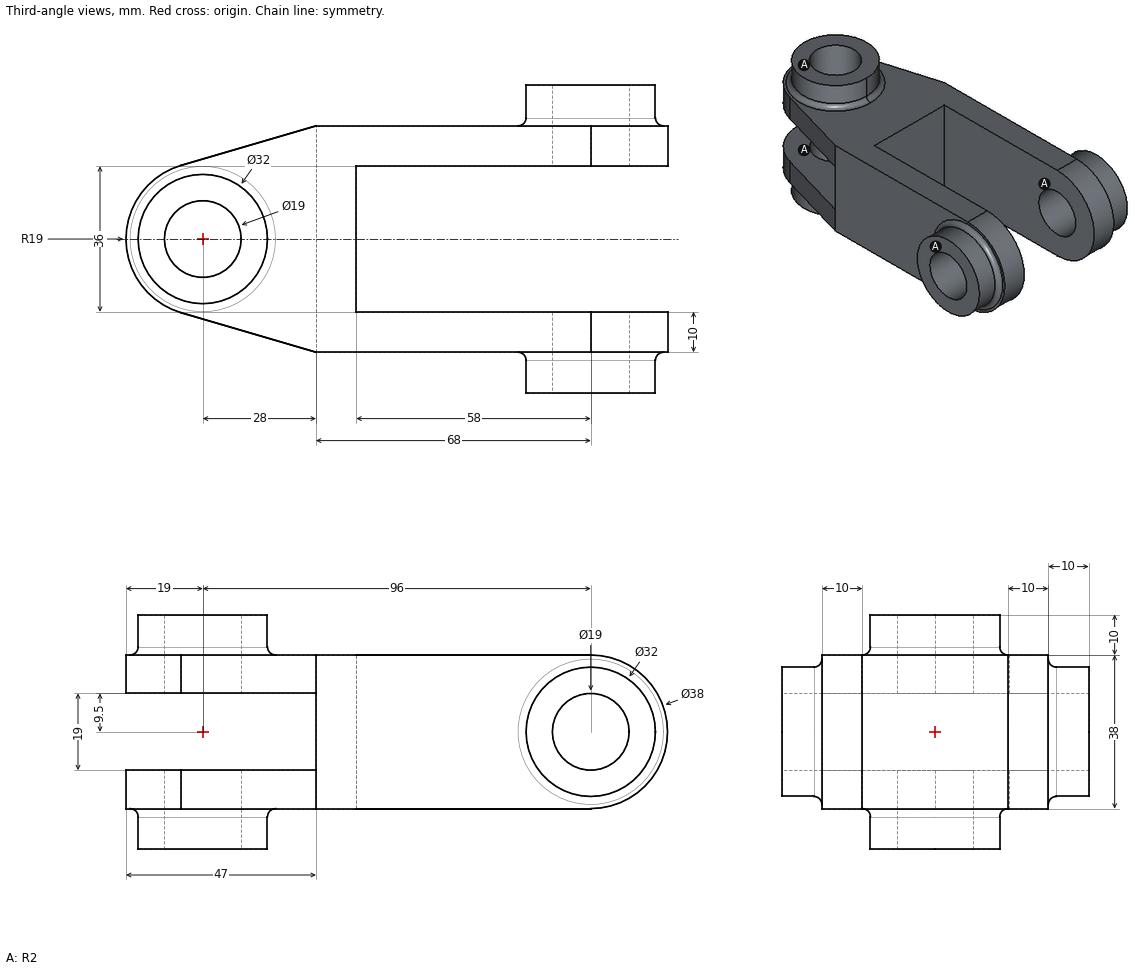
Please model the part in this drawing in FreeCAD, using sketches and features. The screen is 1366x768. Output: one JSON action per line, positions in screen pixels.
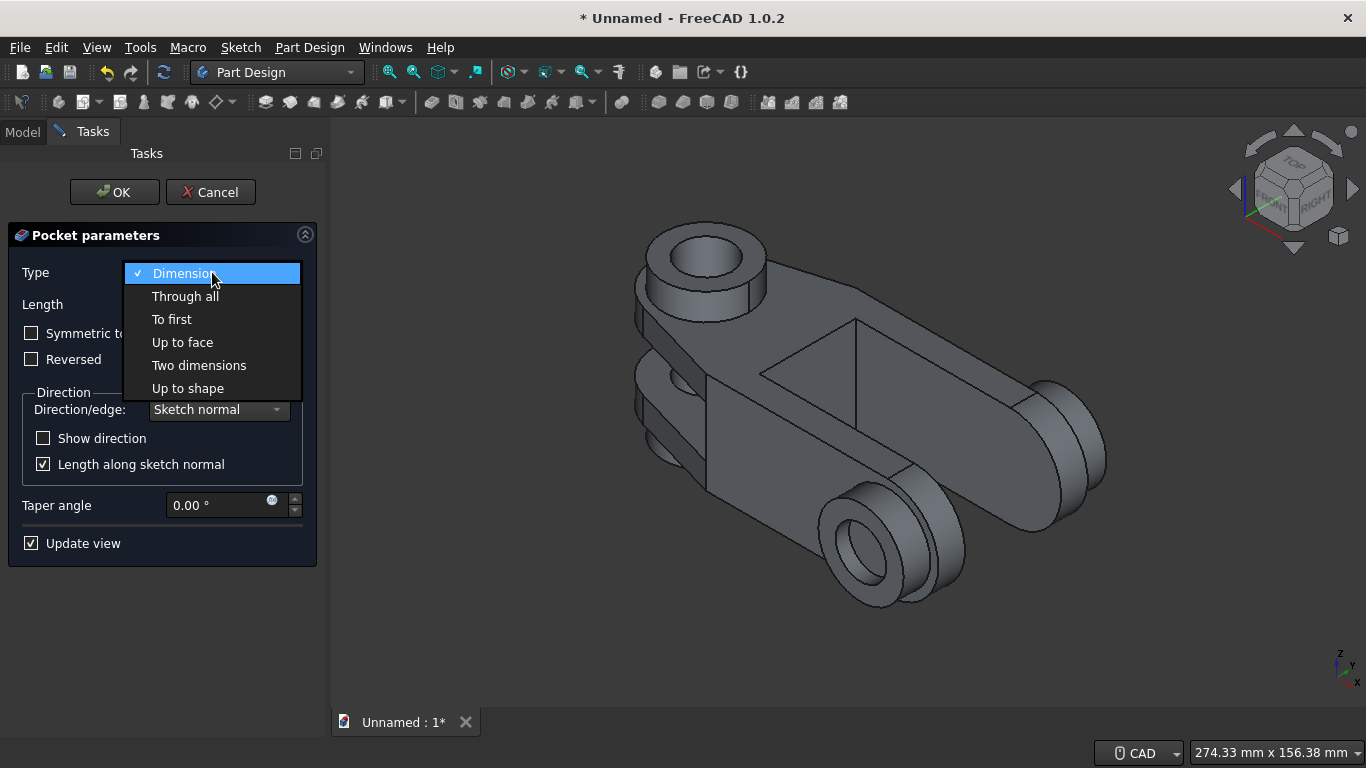
{"action": "left_click", "coordinate": [212, 296]}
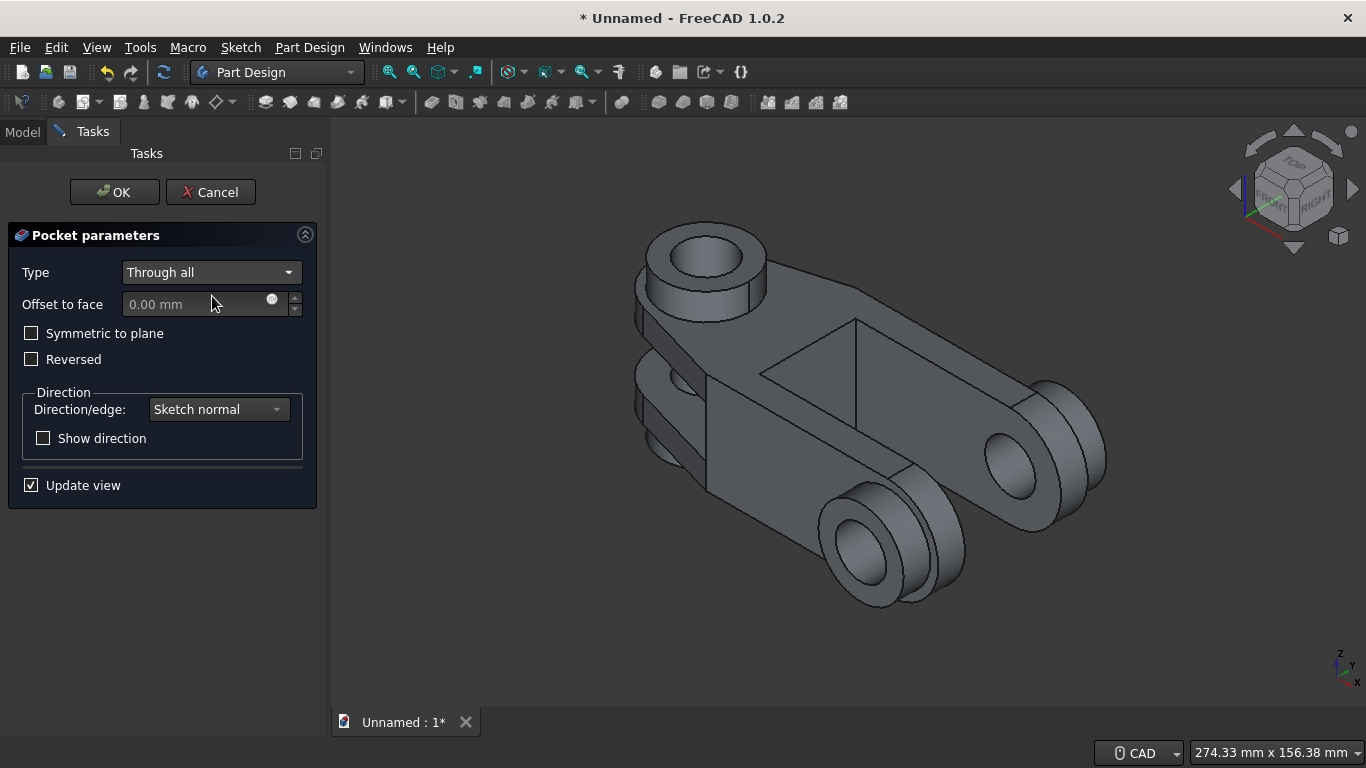
{"action": "left_click", "coordinate": [115, 192]}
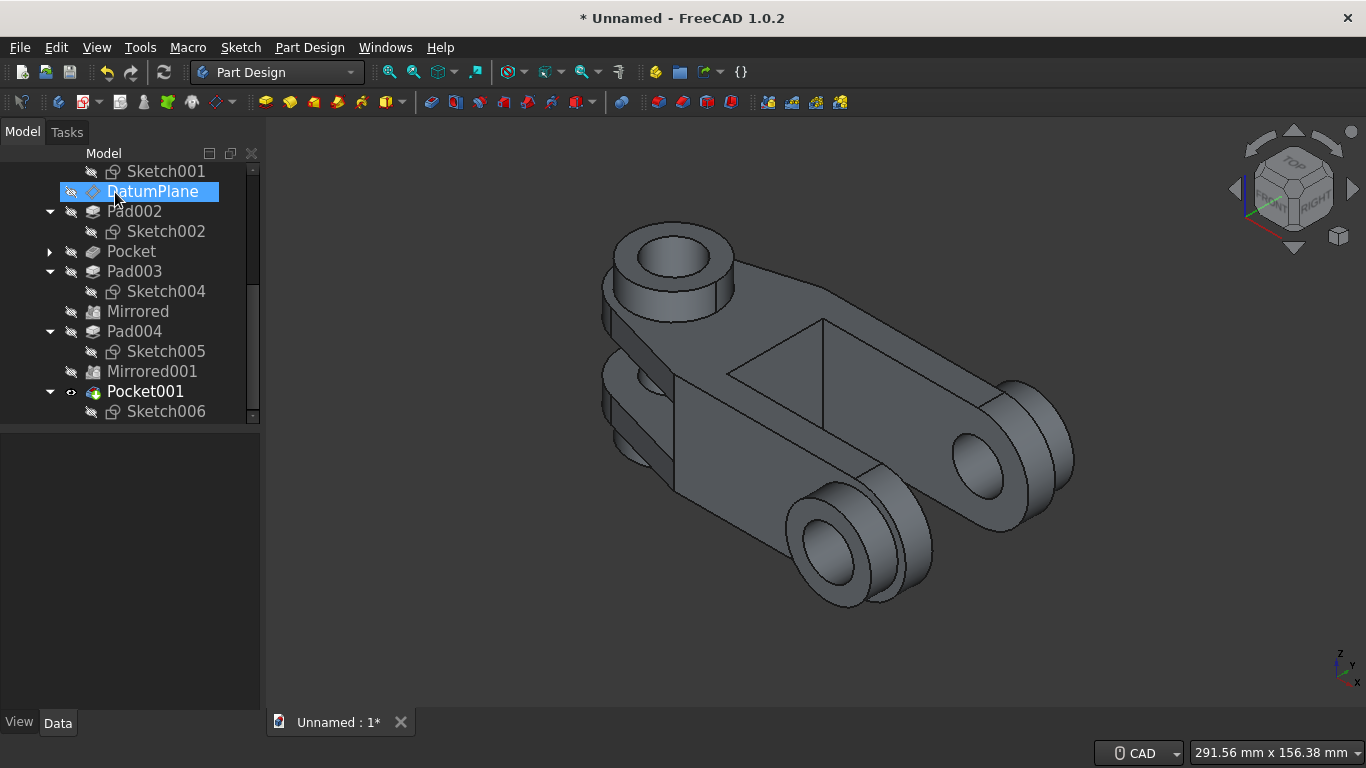
{"action": "key", "text": "2"}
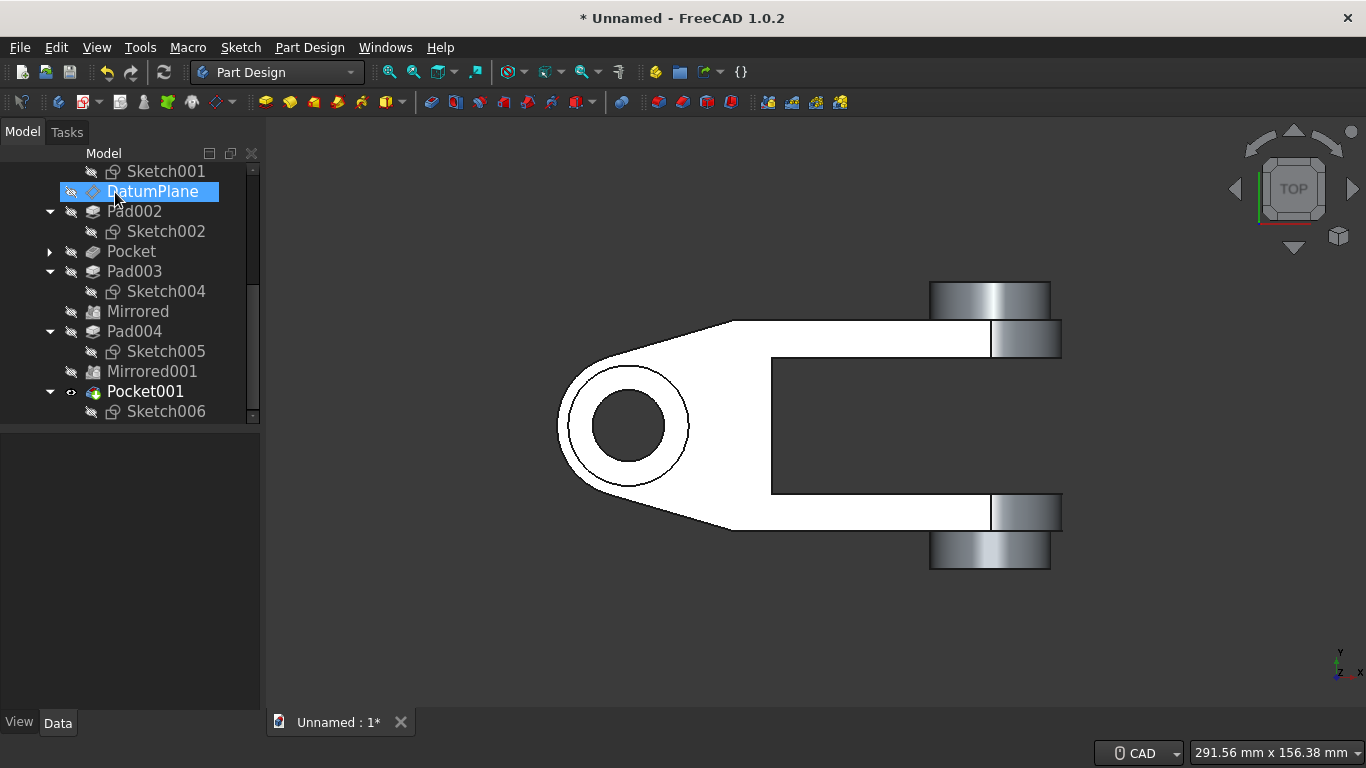
{"action": "key", "text": "0"}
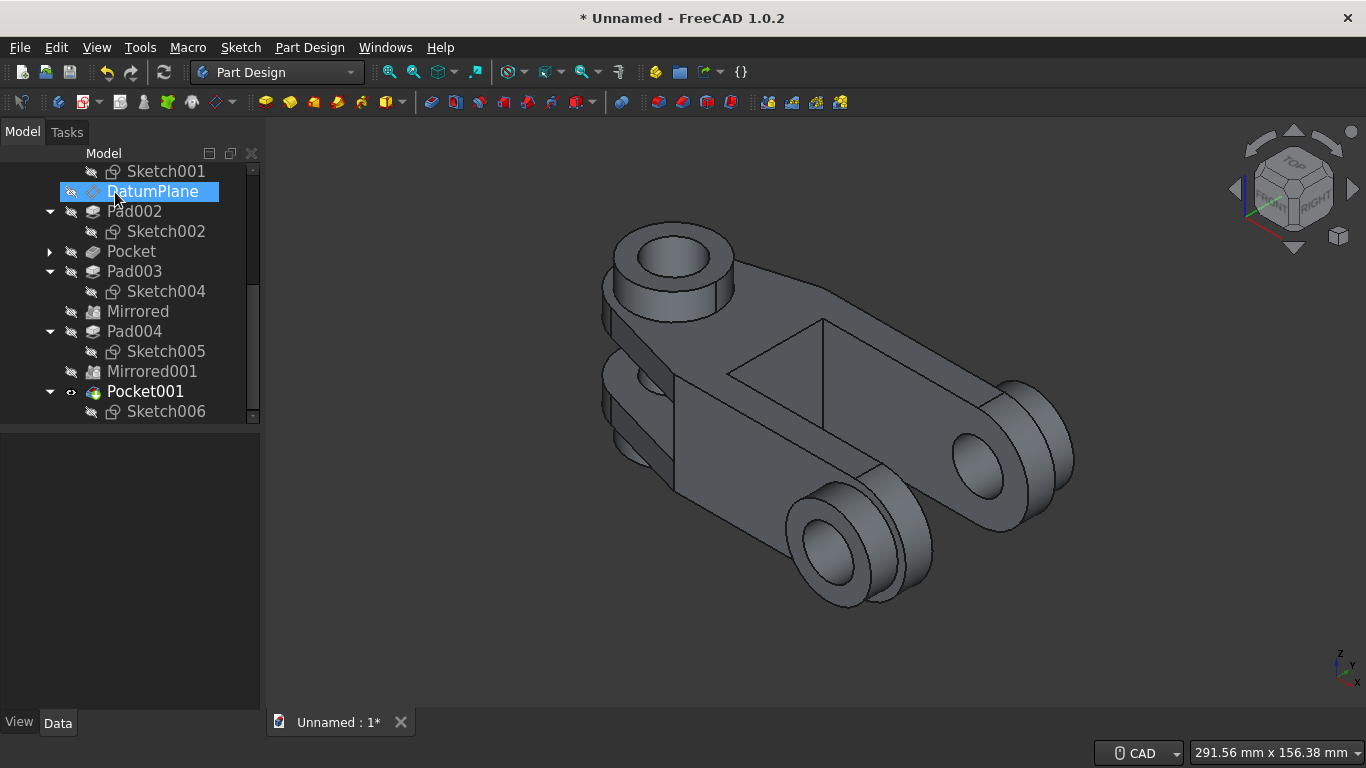
{"action": "key", "text": "1"}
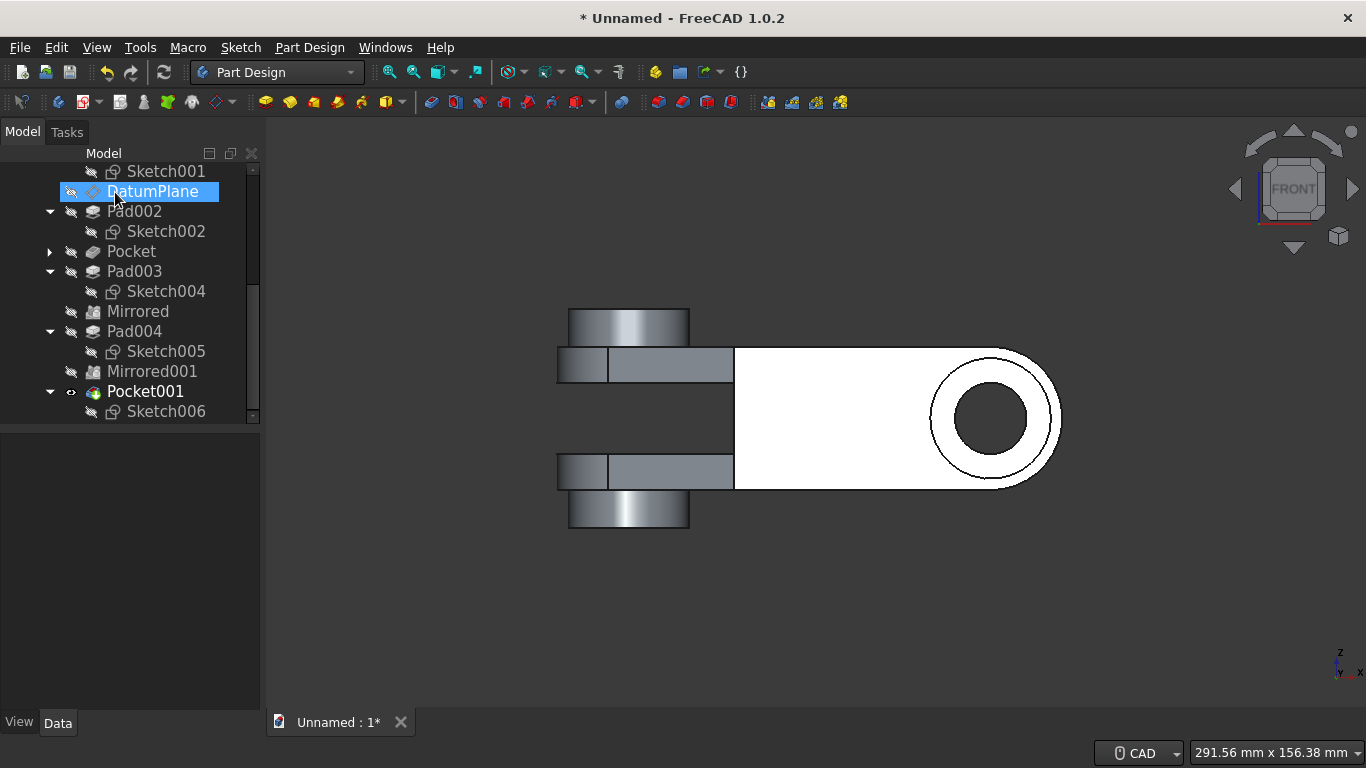
{"action": "key", "text": "3"}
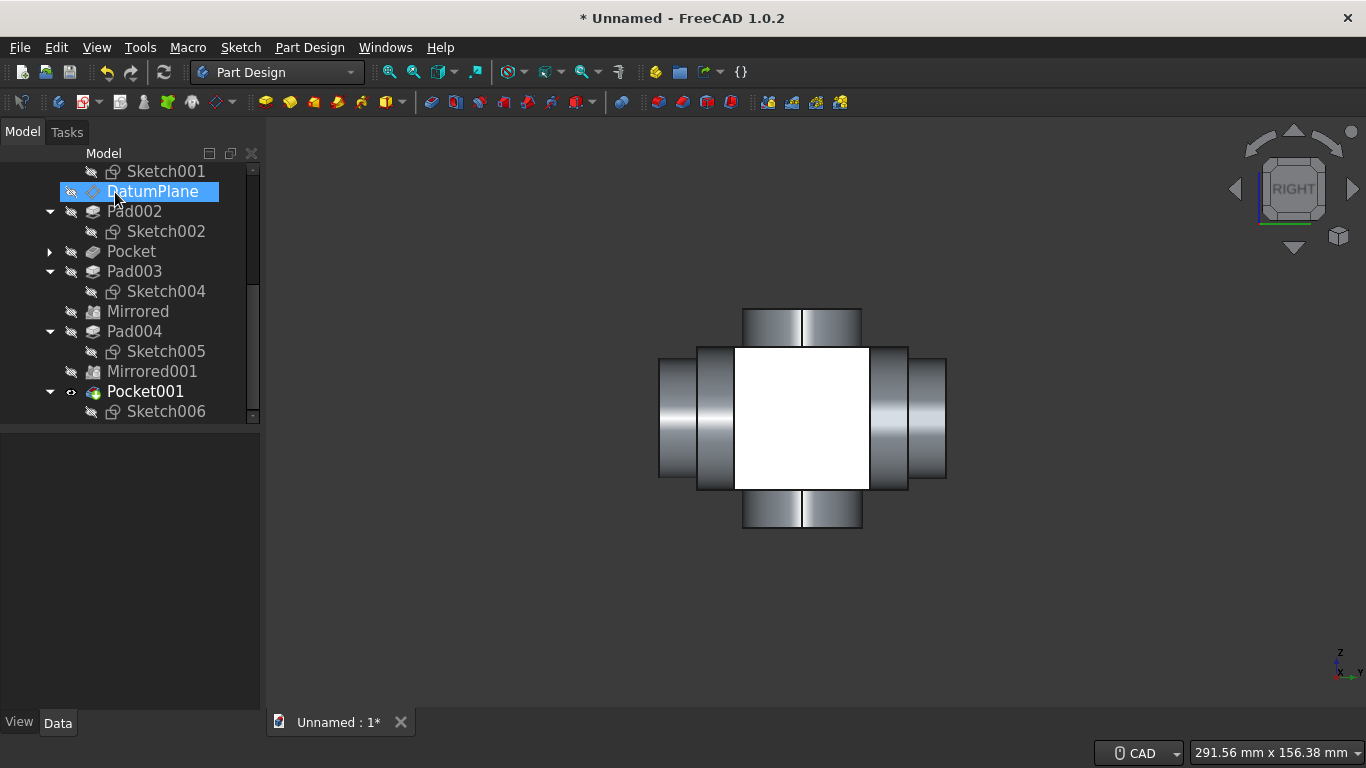
{"action": "left_click", "coordinate": [390, 72]}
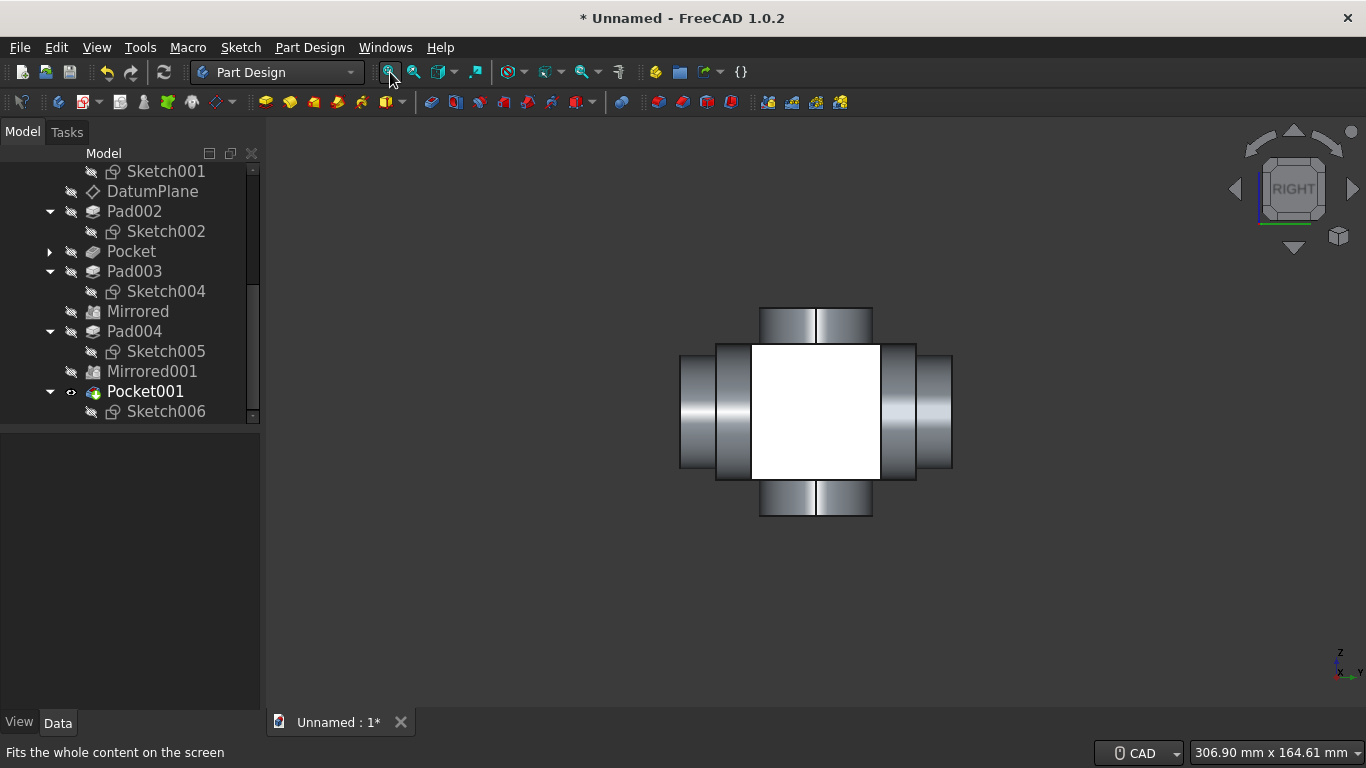
{"action": "key", "text": "5"}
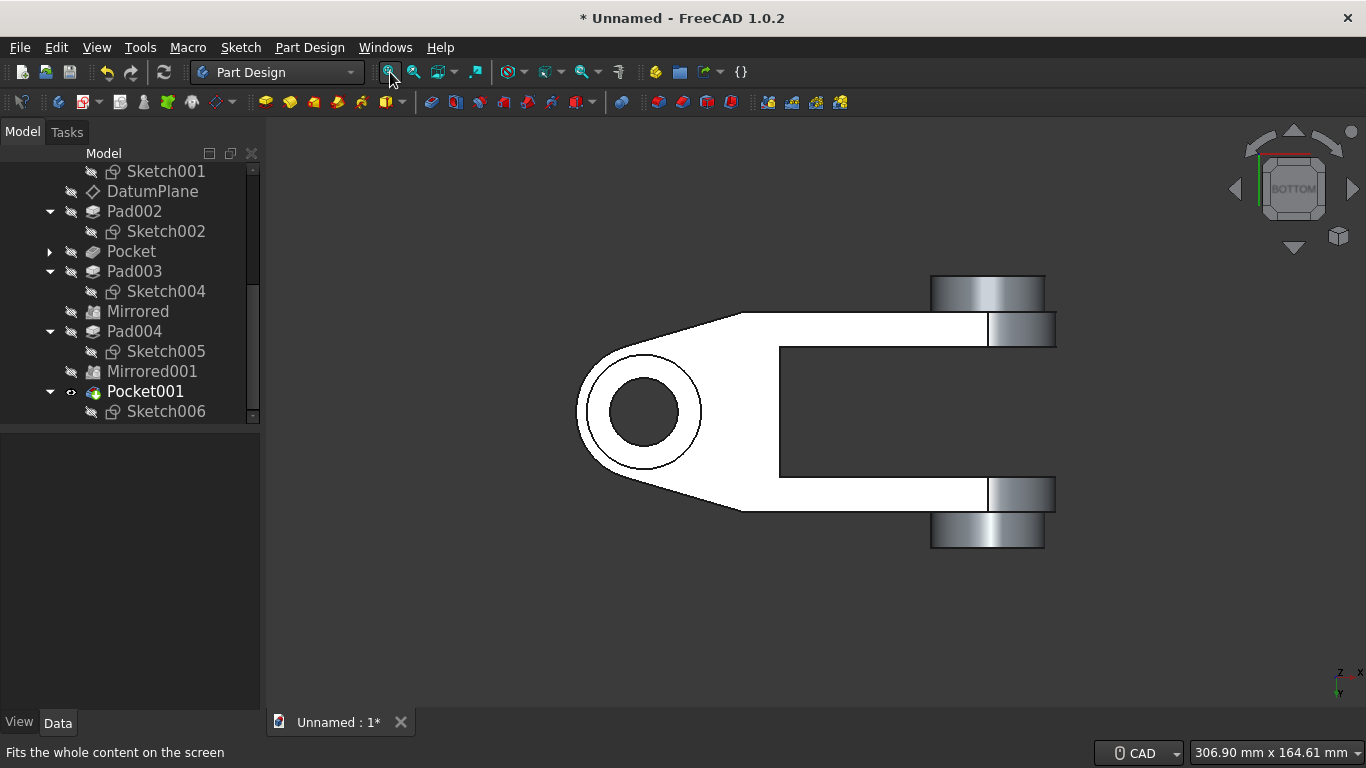
{"action": "key", "text": "4"}